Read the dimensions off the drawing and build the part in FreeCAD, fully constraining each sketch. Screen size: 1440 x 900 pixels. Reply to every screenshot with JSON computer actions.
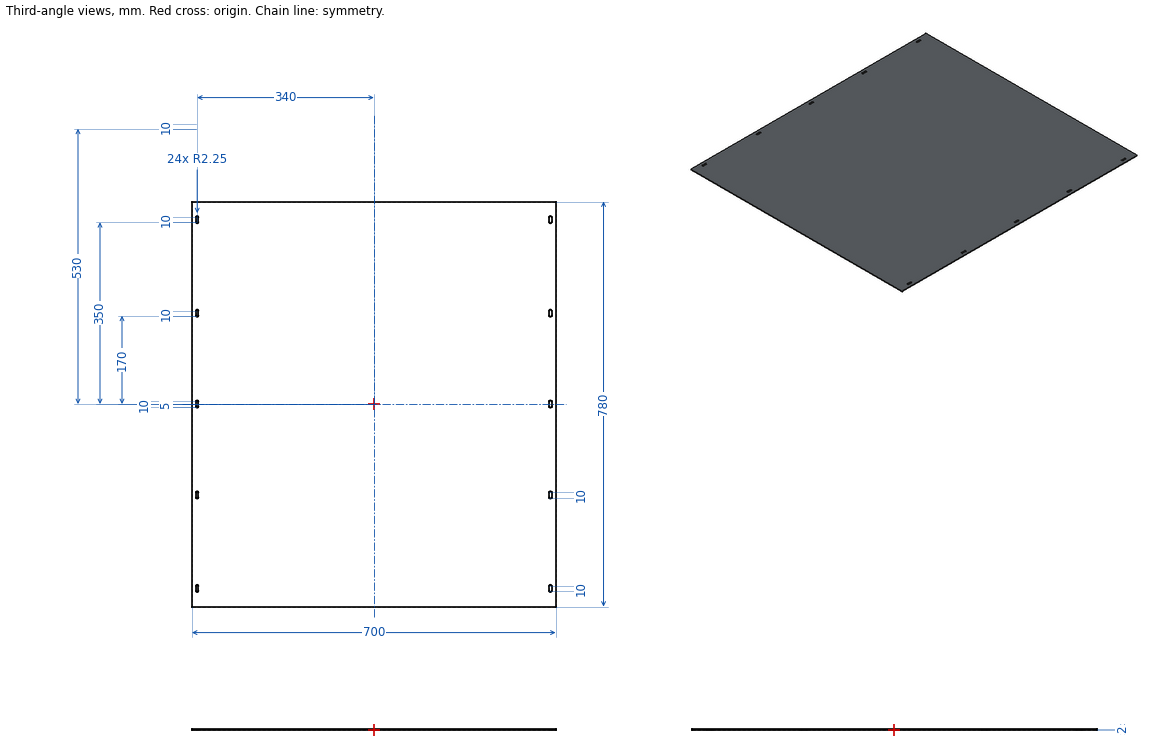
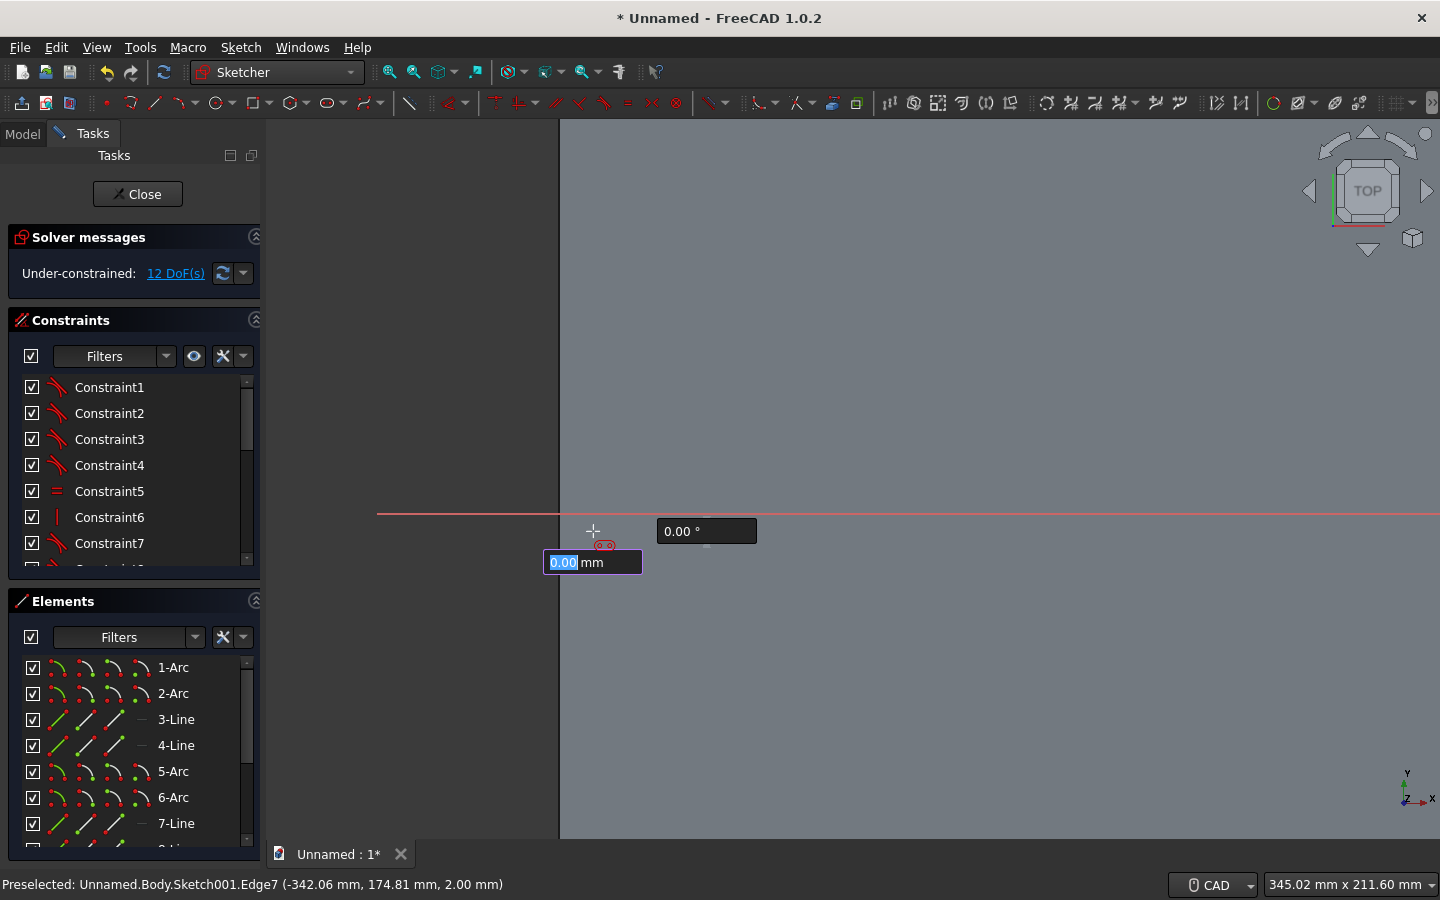
{"action": "left_click", "coordinate": [593, 497]}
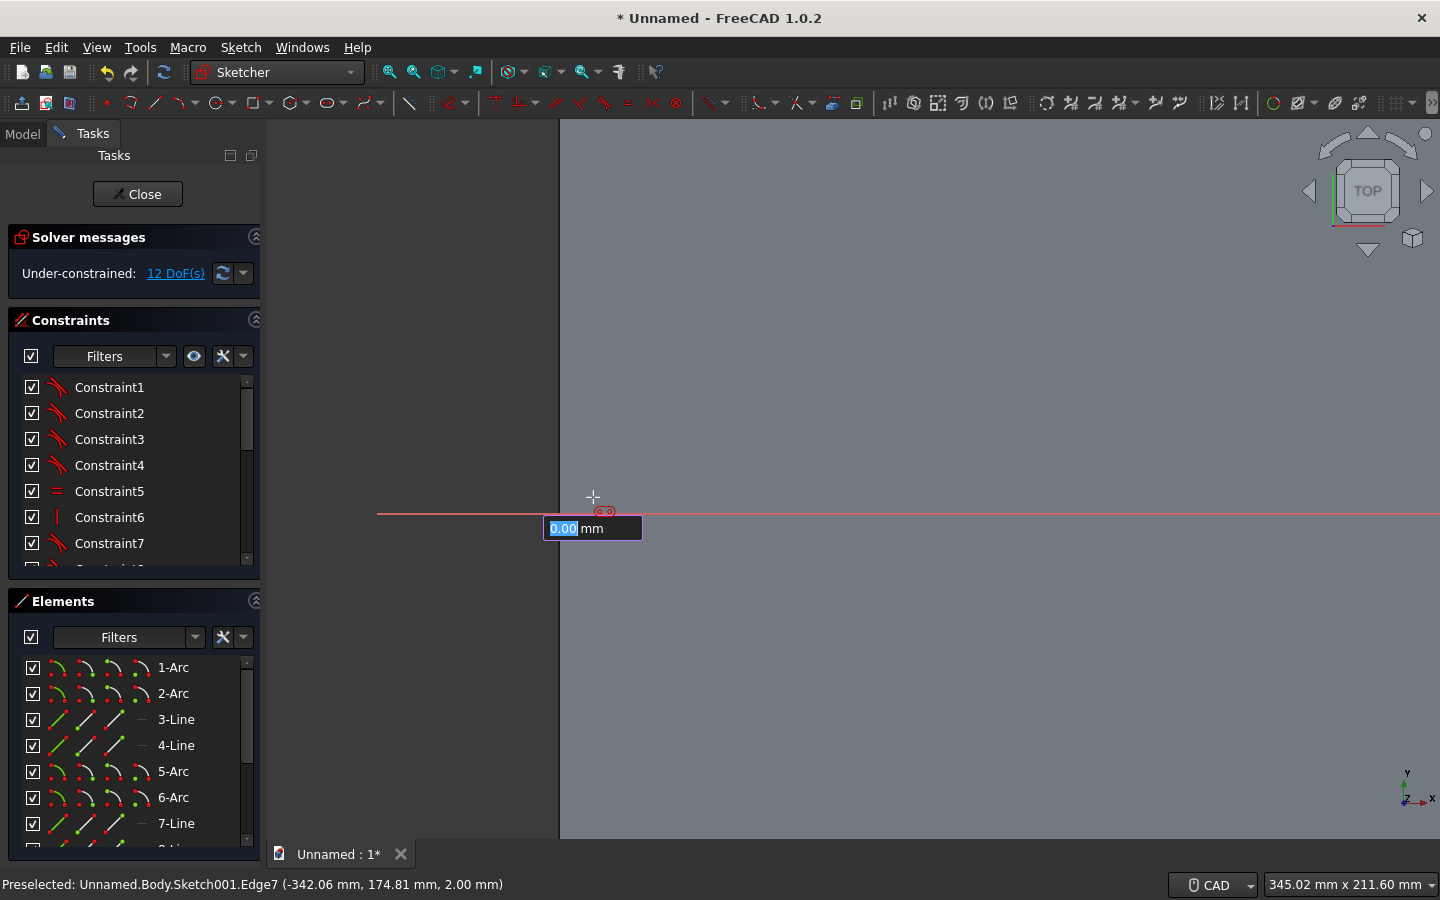
{"action": "scroll", "coordinate": [586, 509], "scroll_direction": "up", "scroll_amount": 6}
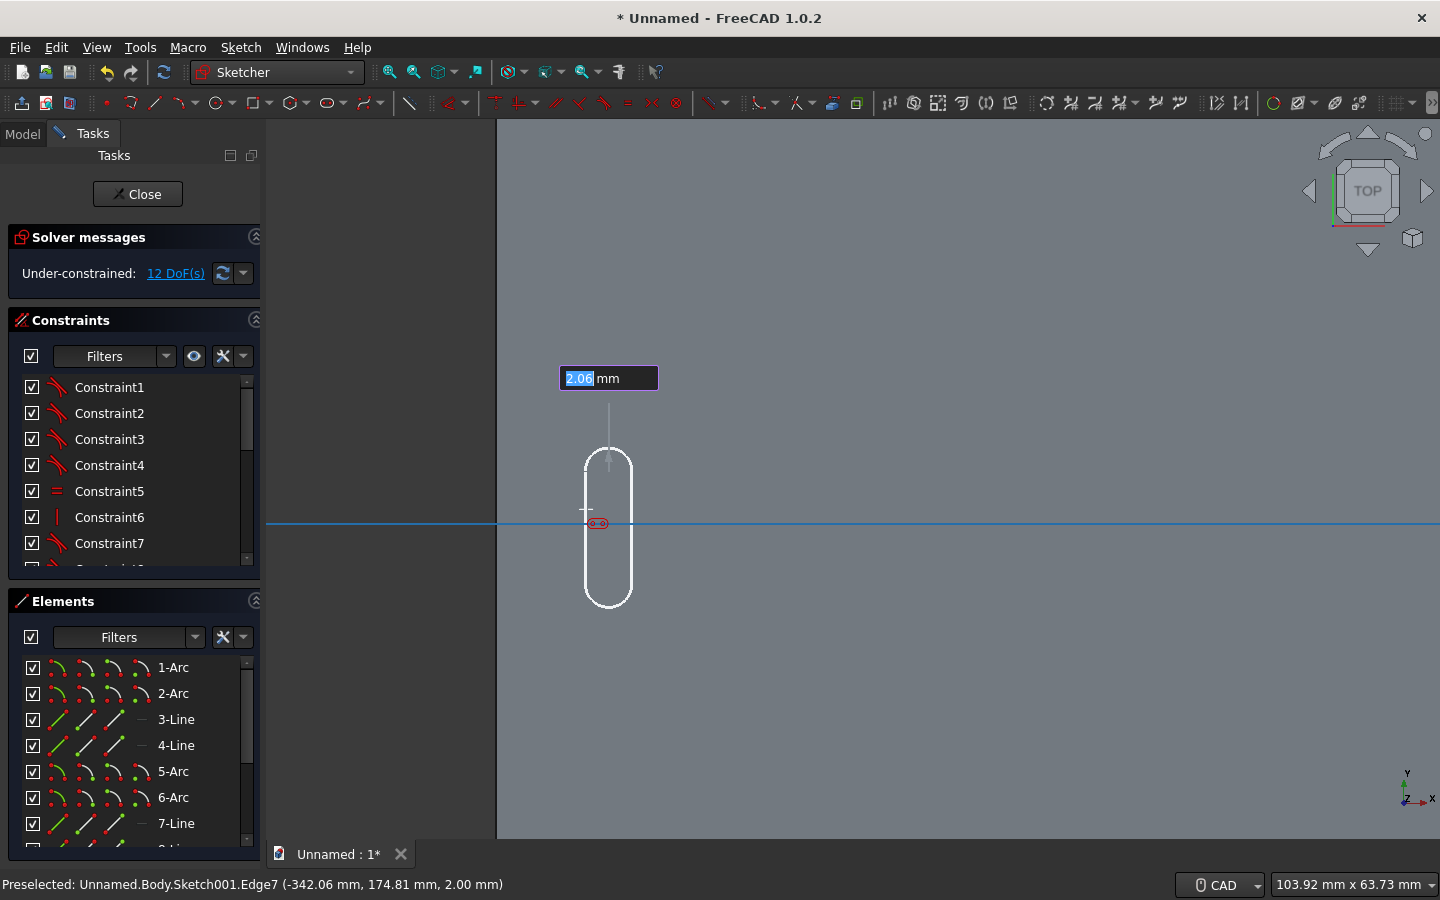
{"action": "left_click", "coordinate": [584, 507]}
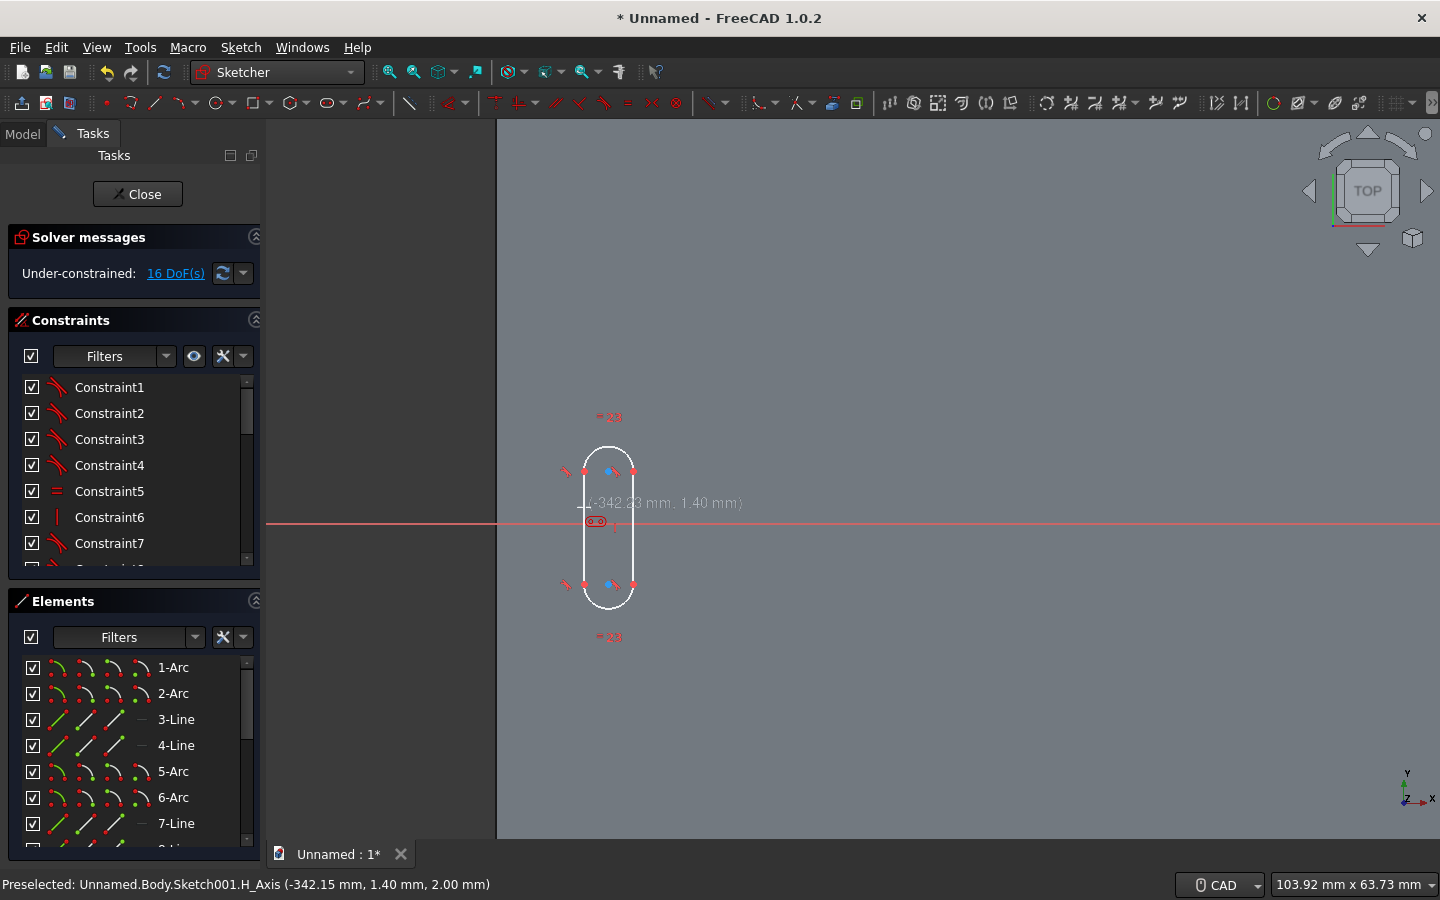
{"action": "scroll", "coordinate": [592, 530], "scroll_direction": "down", "scroll_amount": 15}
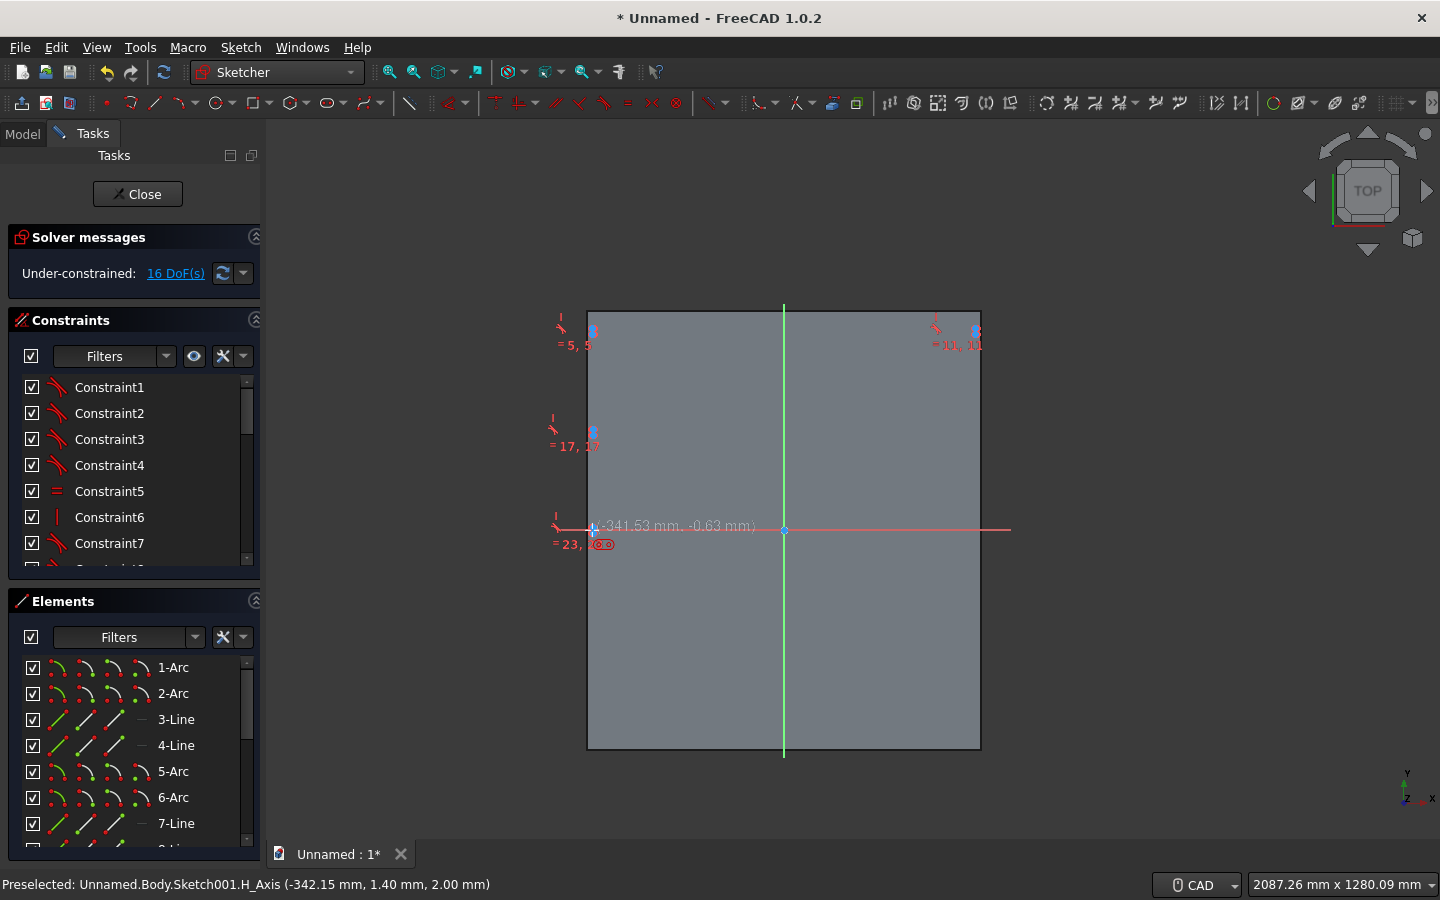
{"action": "scroll", "coordinate": [976, 435], "scroll_direction": "up", "scroll_amount": 15}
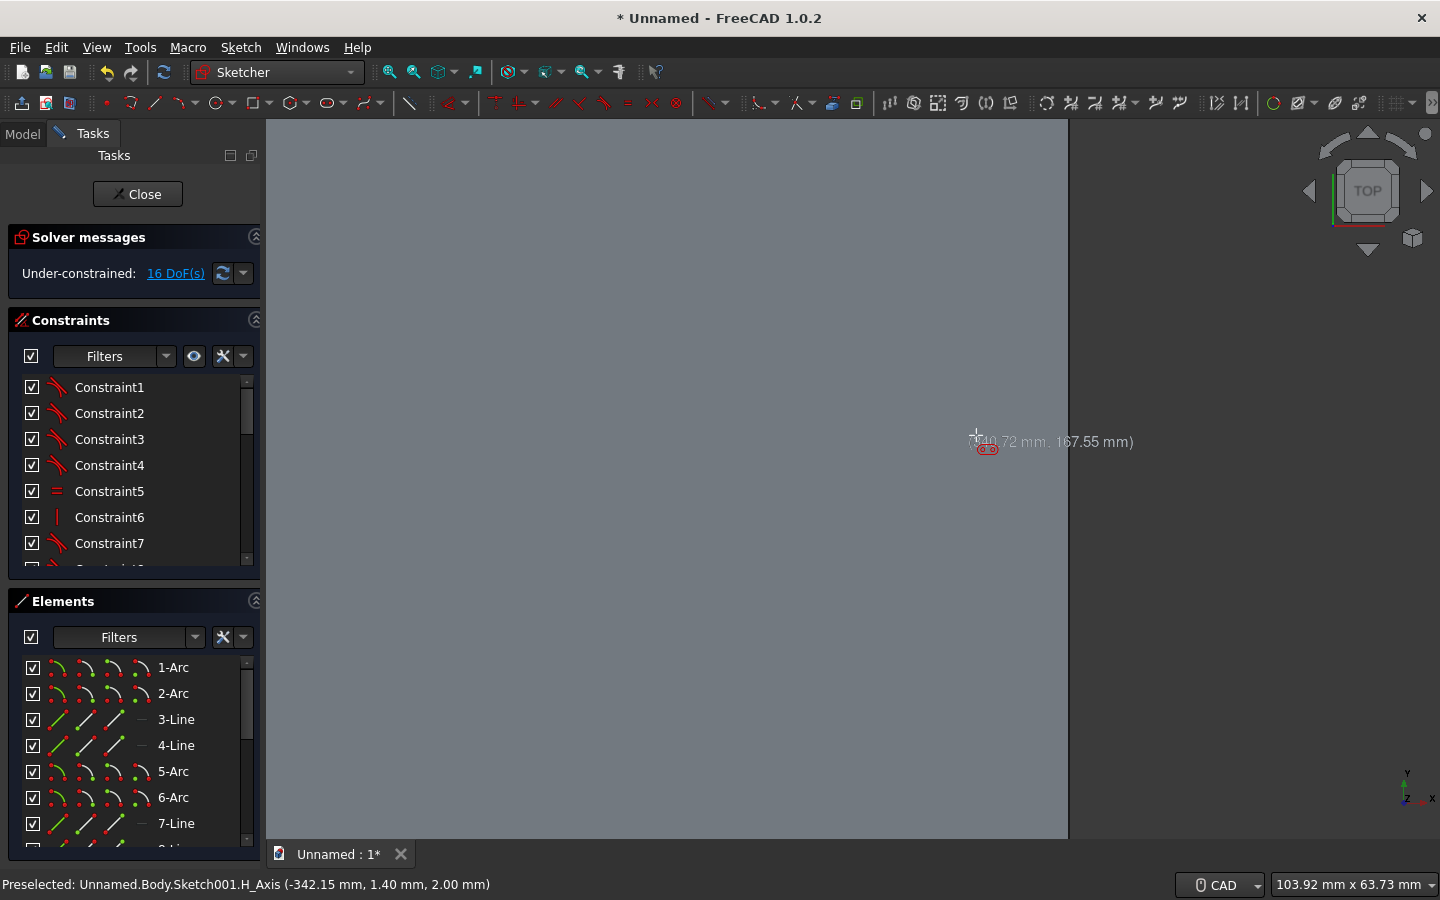
{"action": "scroll", "coordinate": [977, 435], "scroll_direction": "down", "scroll_amount": 15}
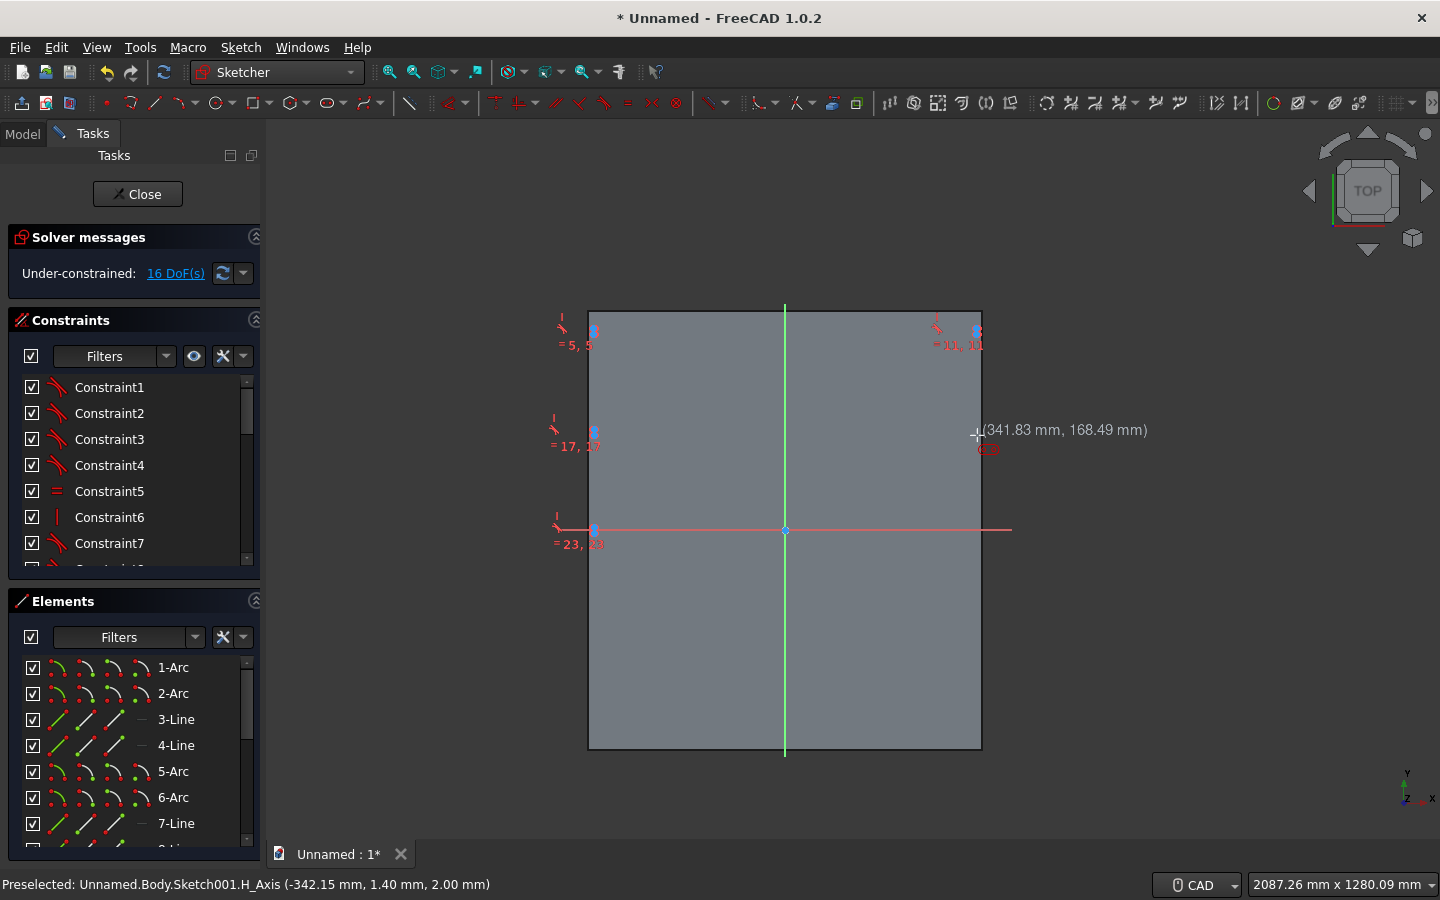
{"action": "left_click", "coordinate": [977, 435]}